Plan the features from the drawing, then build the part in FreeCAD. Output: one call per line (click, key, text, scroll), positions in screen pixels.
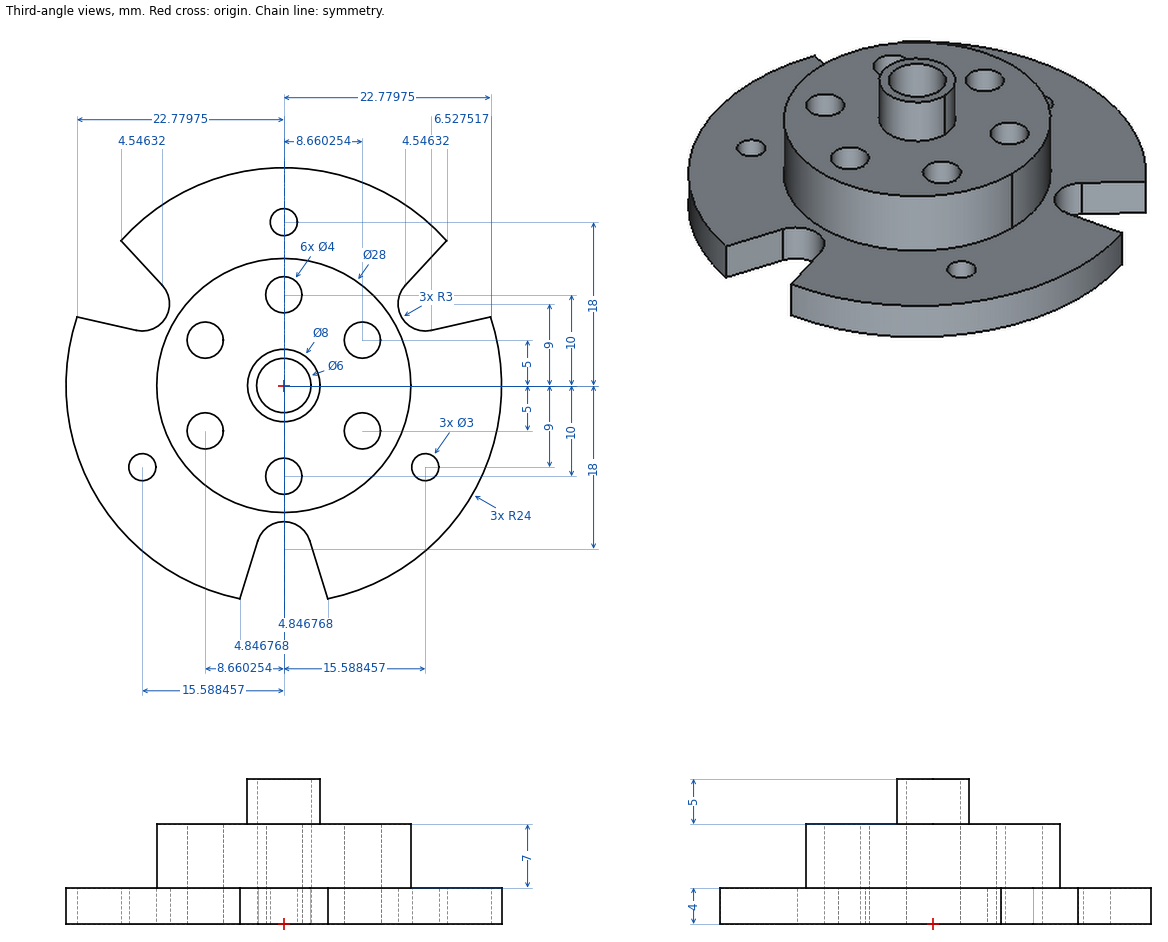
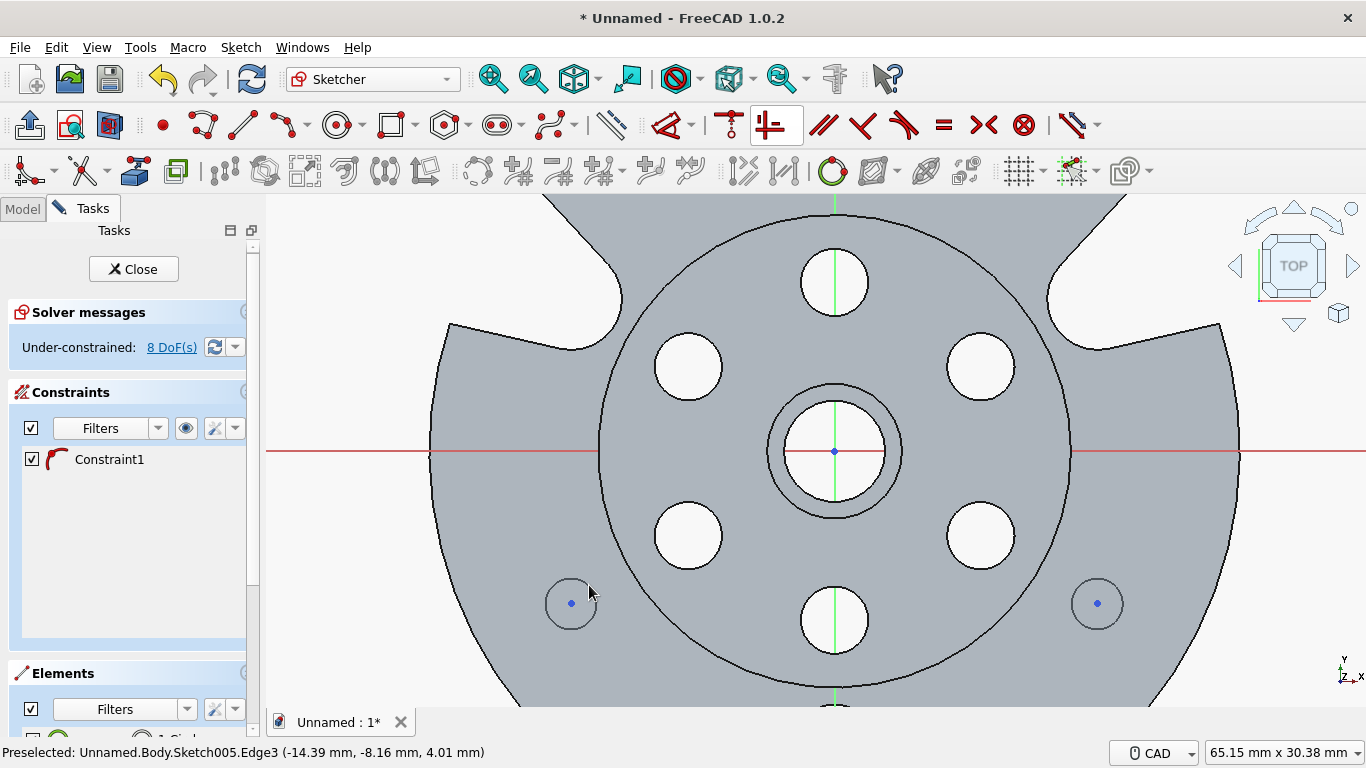
click(1115, 586)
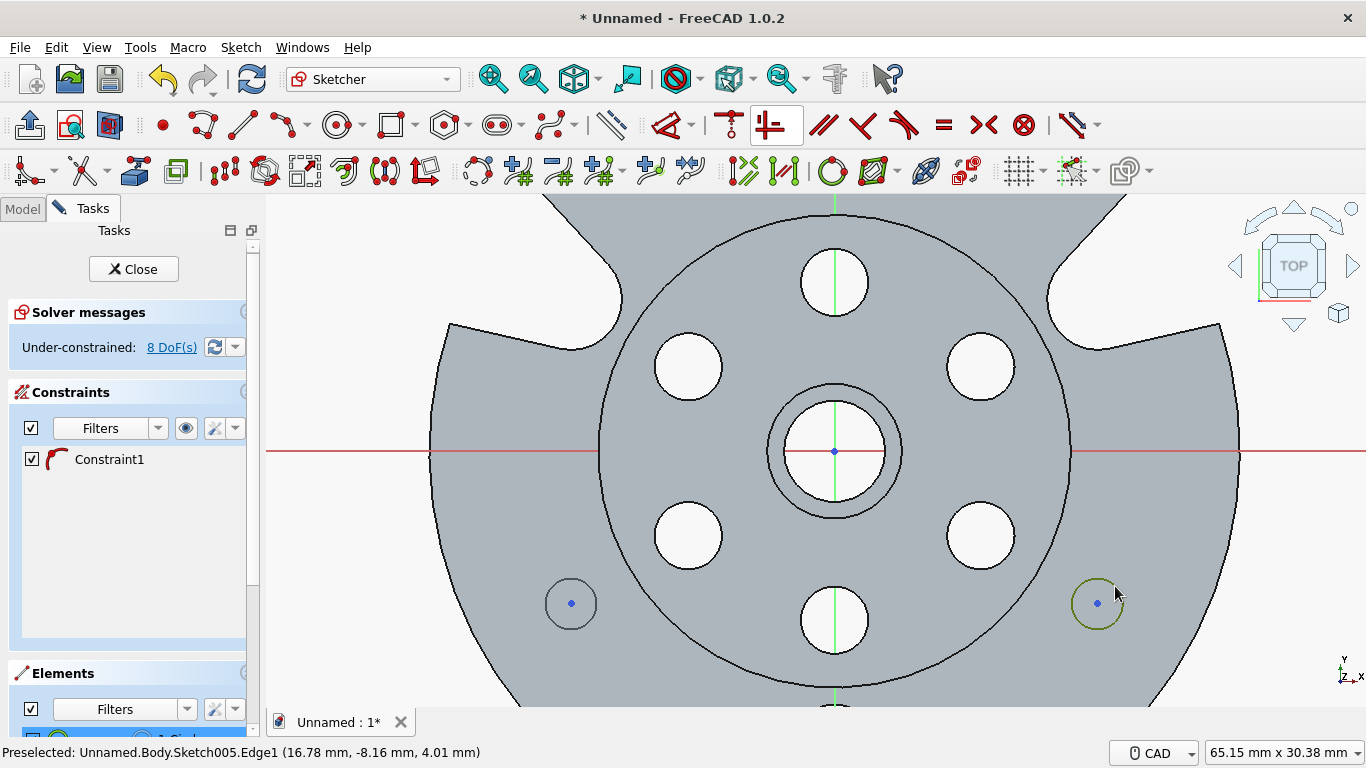
scroll(570, 603, down, 2)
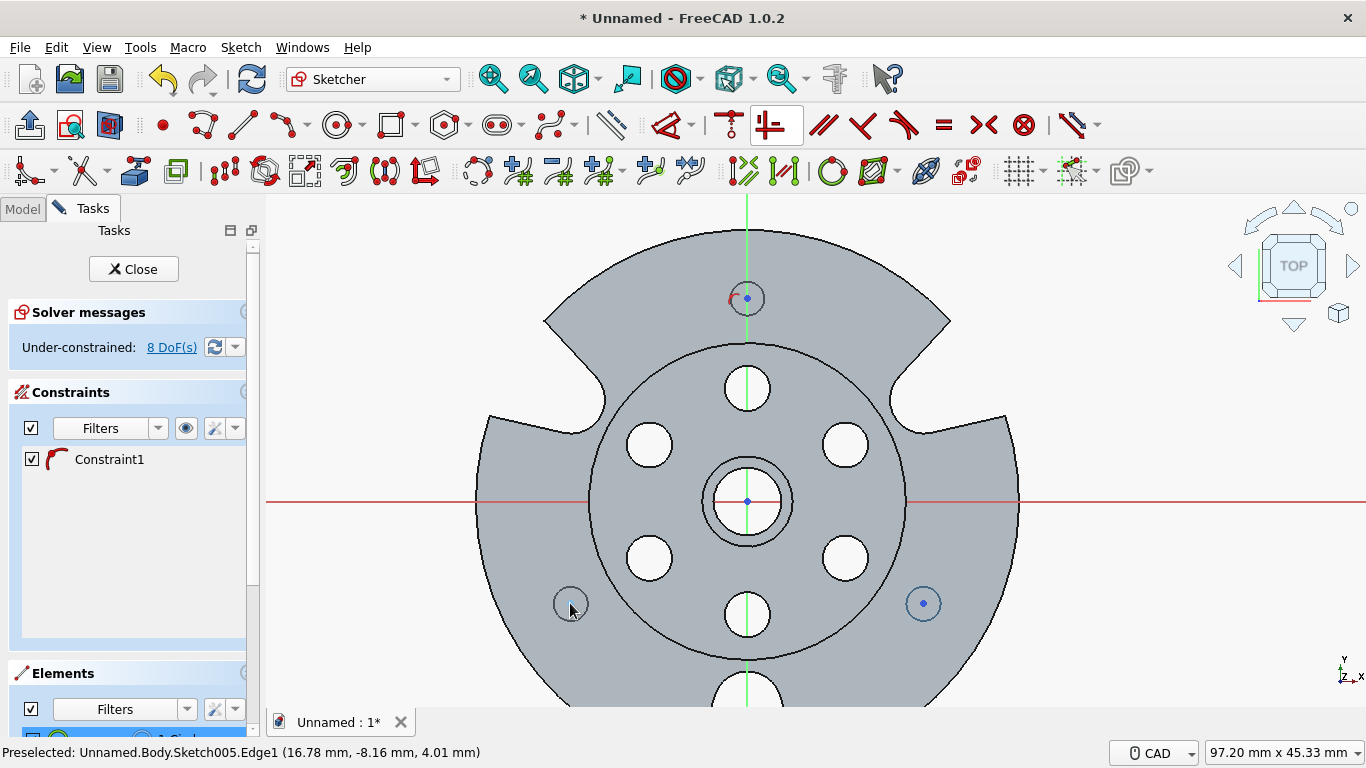
click(759, 287)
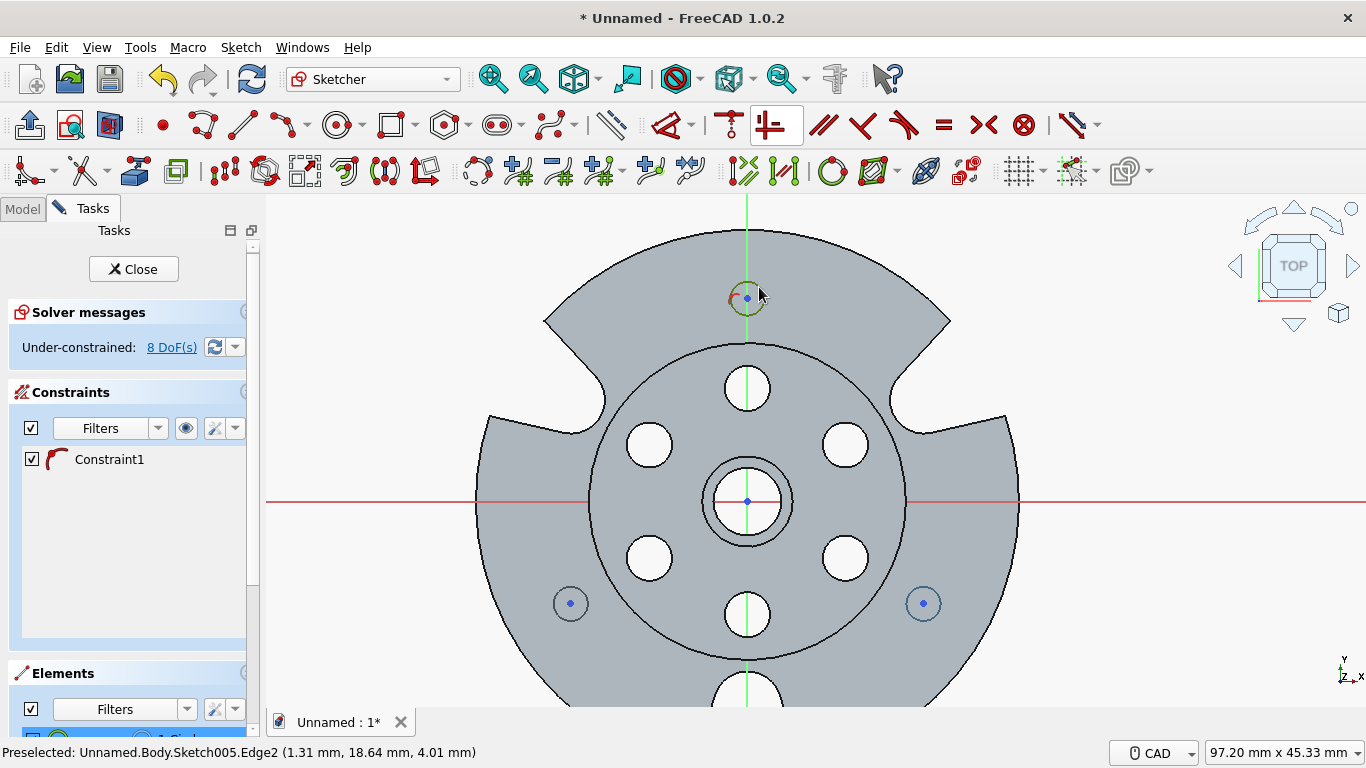
click(583, 592)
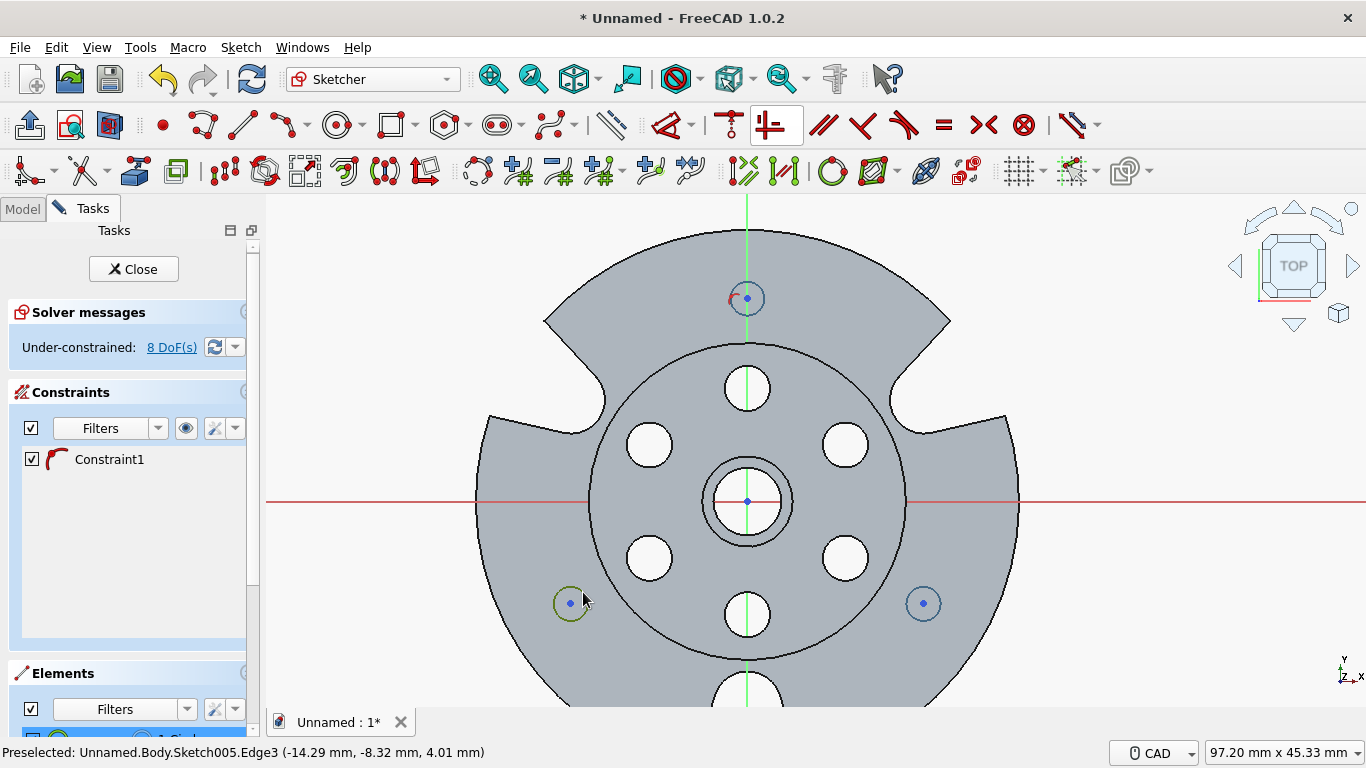
key(e)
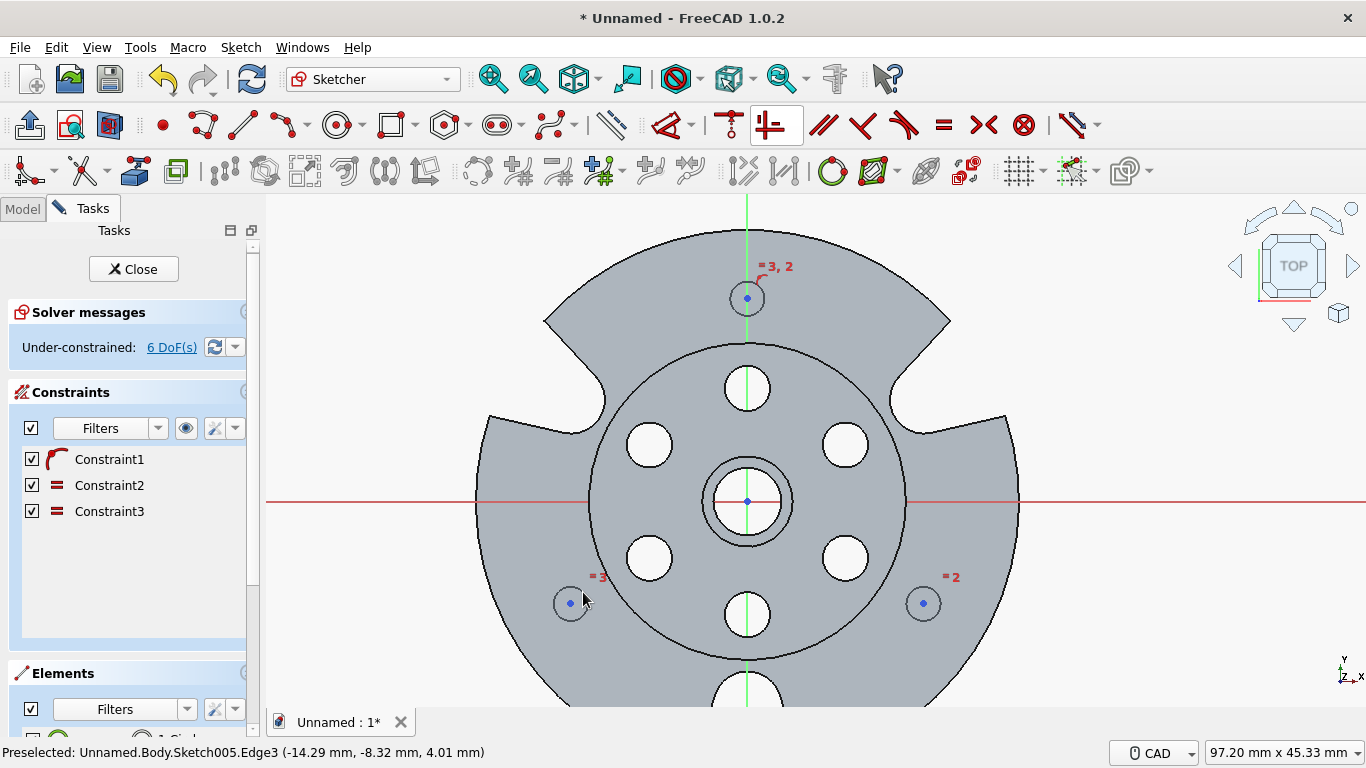
click(924, 604)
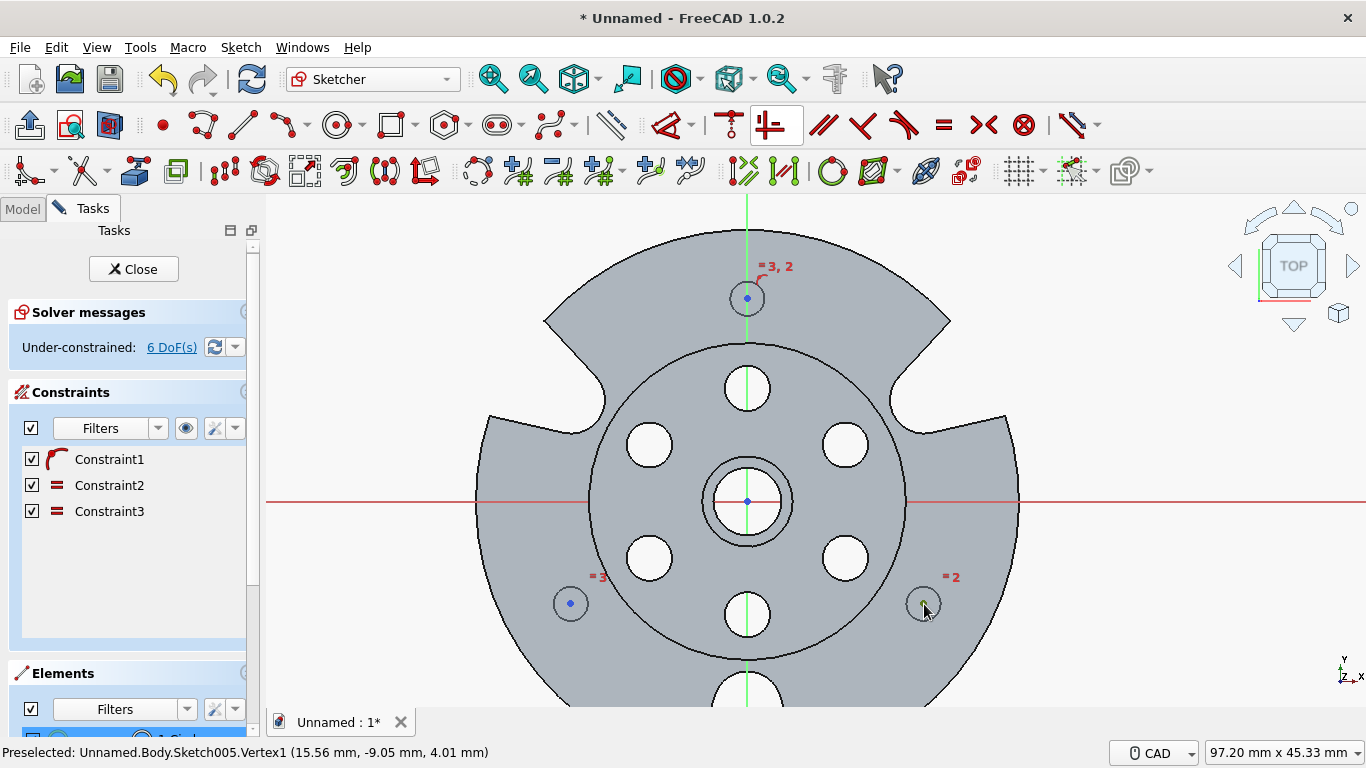
click(571, 604)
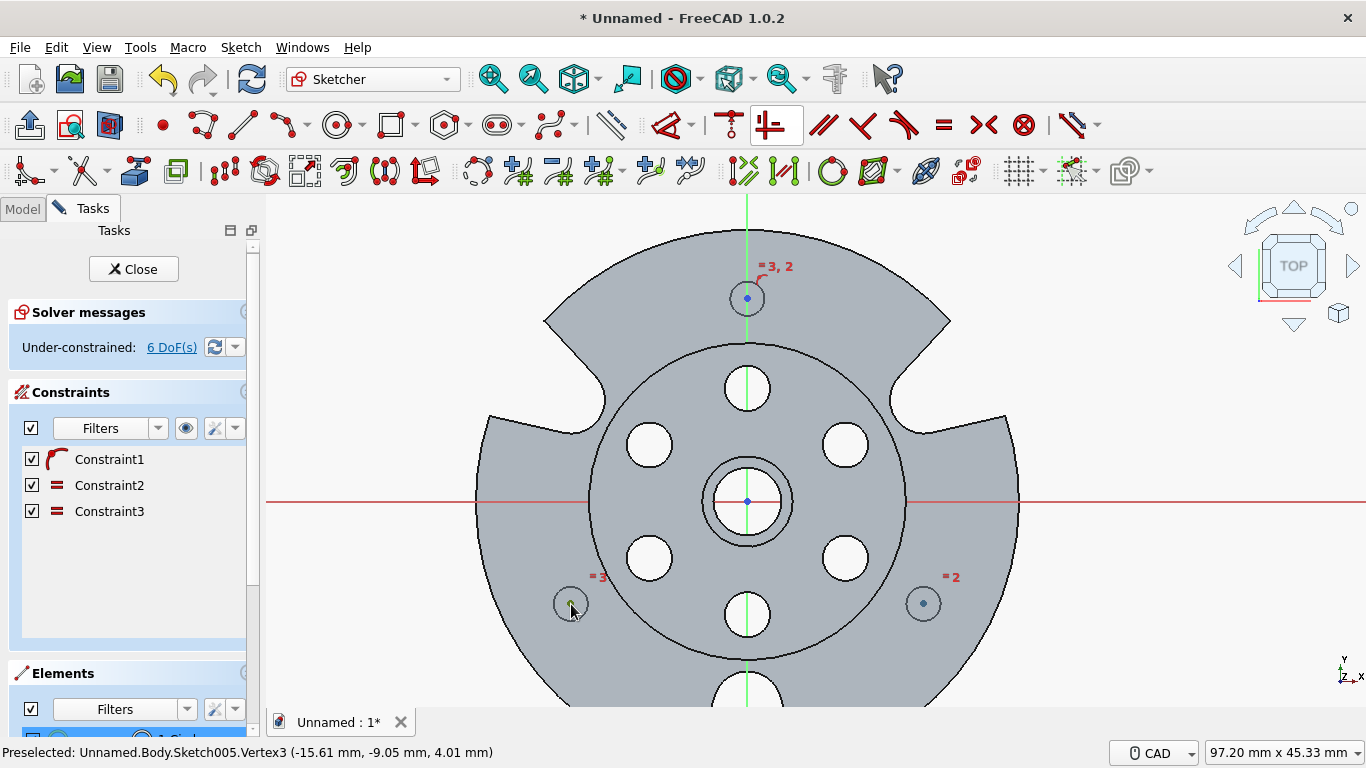
key(h)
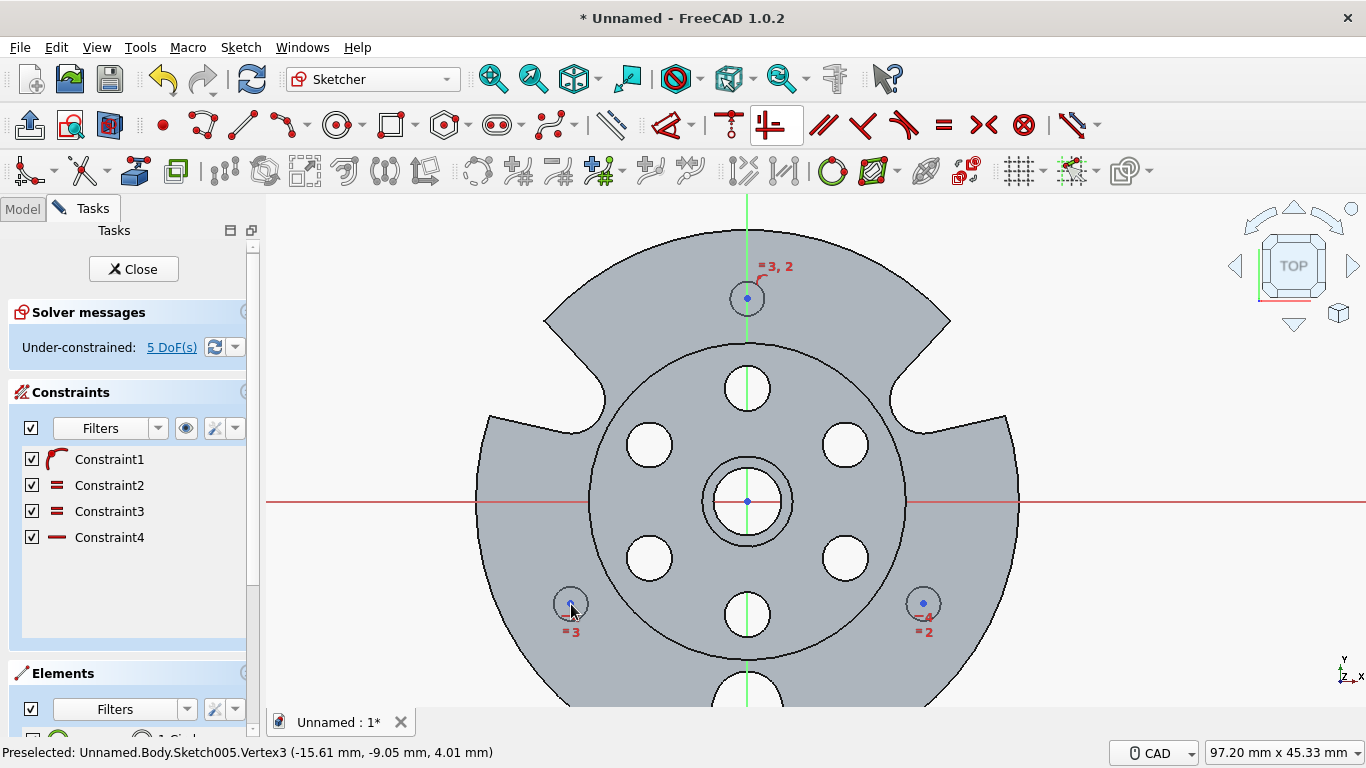
key(d)